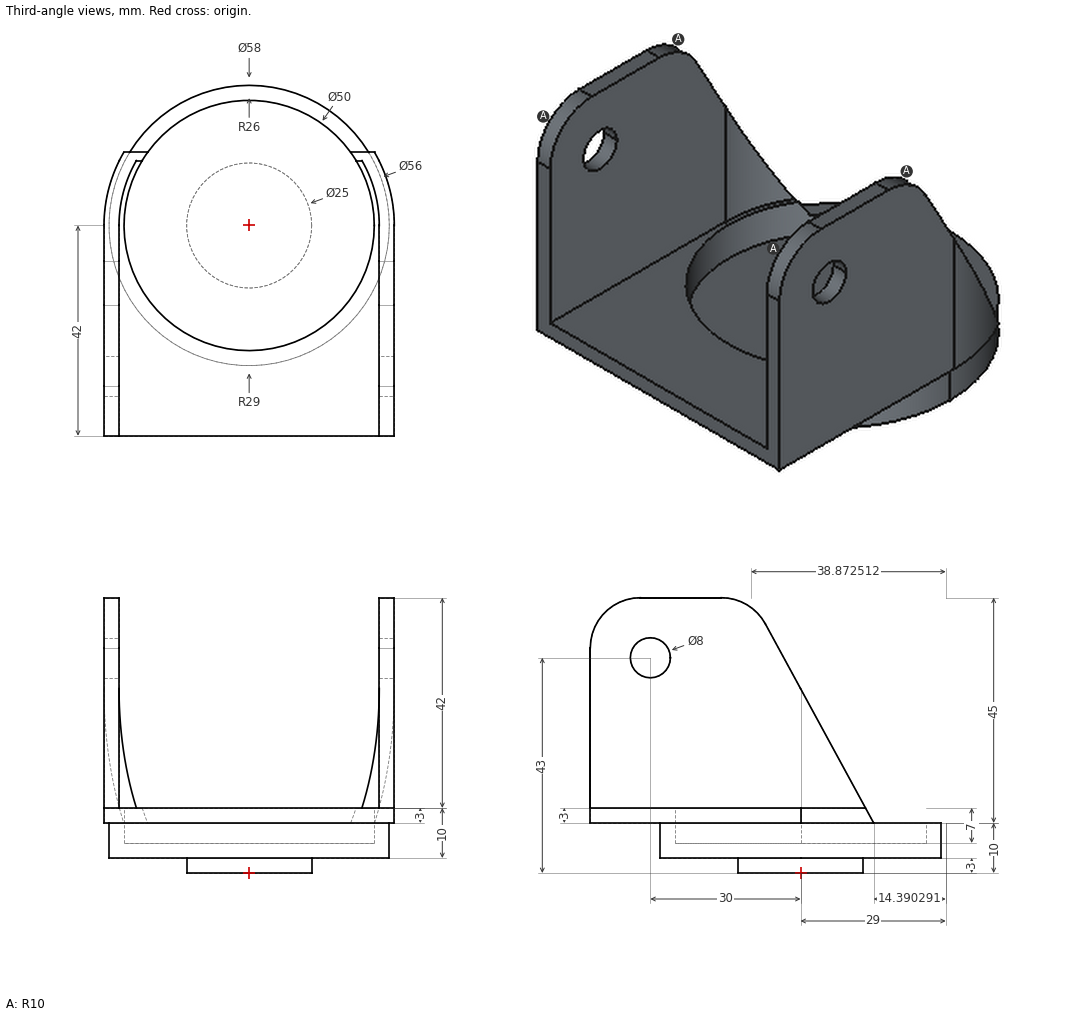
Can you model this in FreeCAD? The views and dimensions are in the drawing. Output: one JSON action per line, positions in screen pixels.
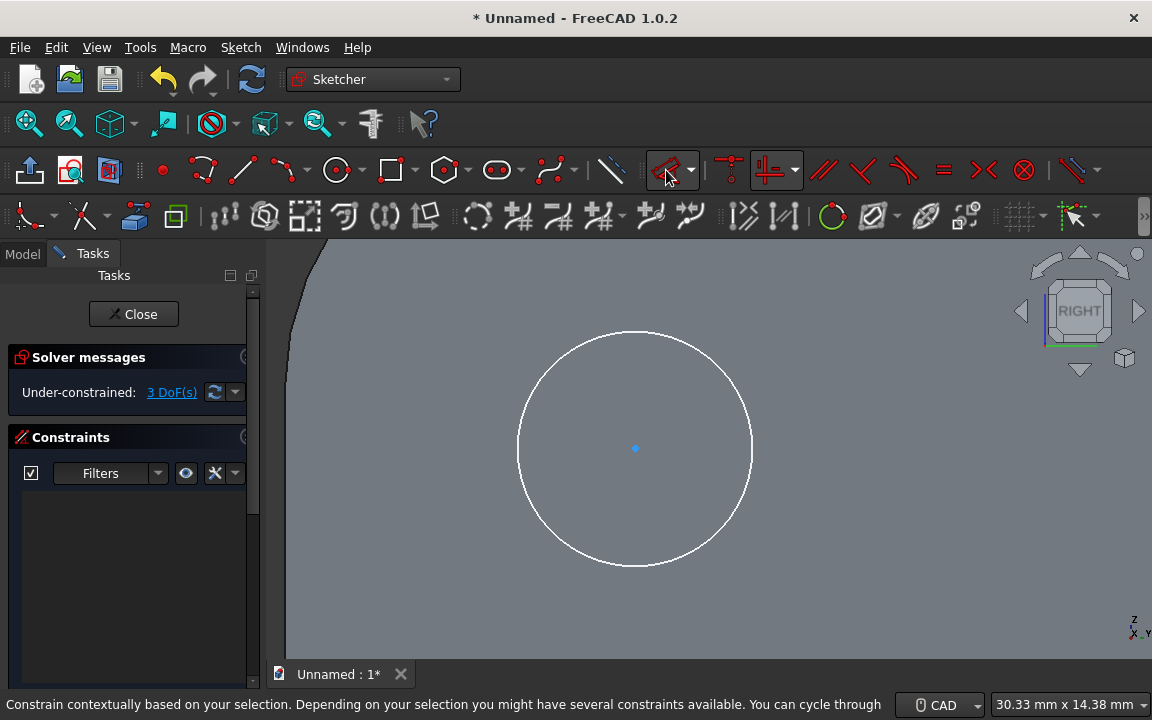
{"action": "left_click", "coordinate": [718, 366]}
{"action": "left_click", "coordinate": [741, 343]}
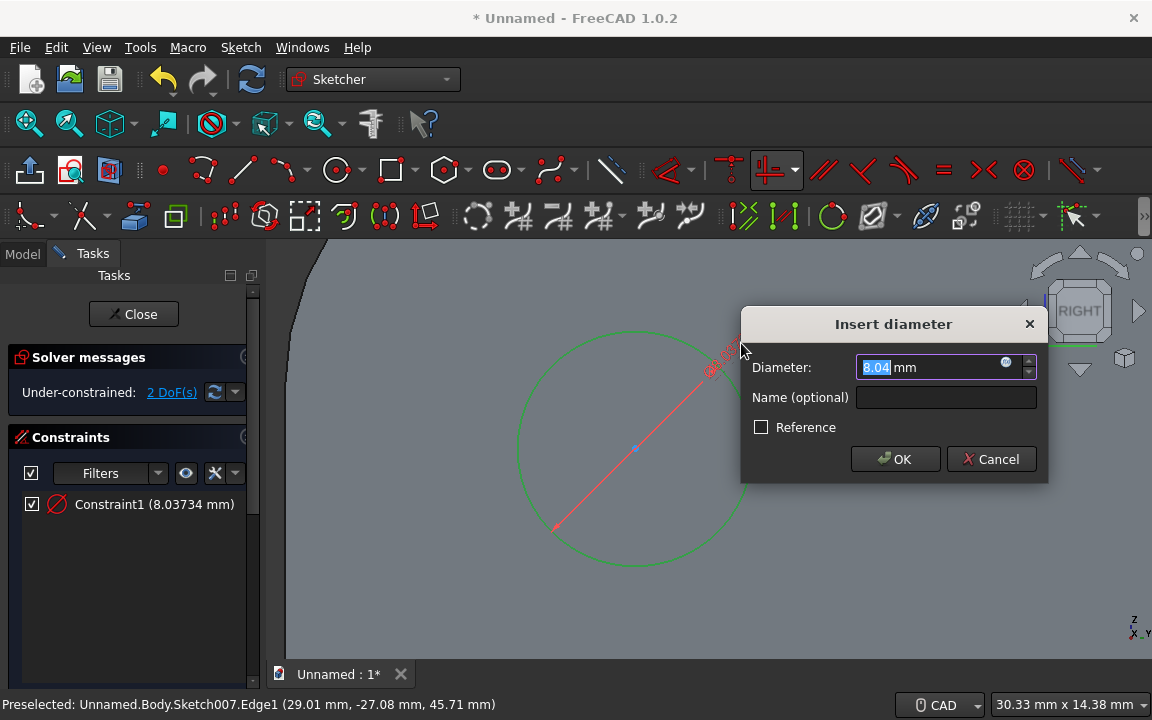
{"action": "type", "text": "8"}
{"action": "key", "text": "Return"}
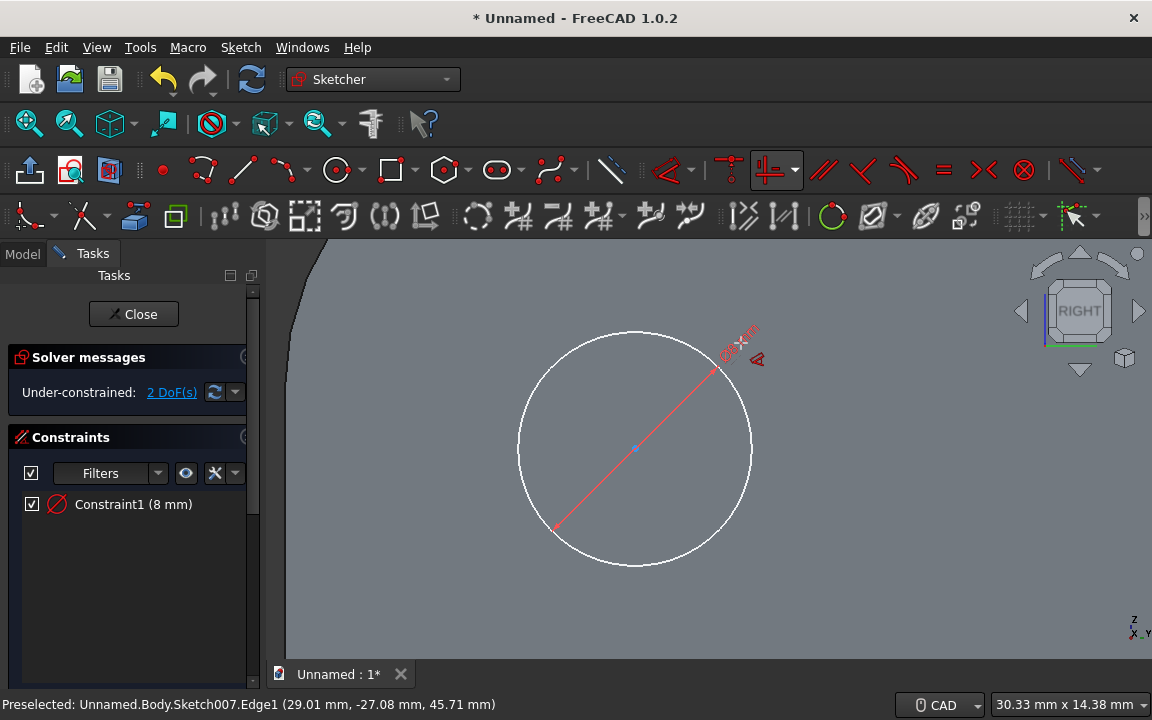
{"action": "left_click", "coordinate": [635, 449]}
{"action": "left_click", "coordinate": [811, 415]}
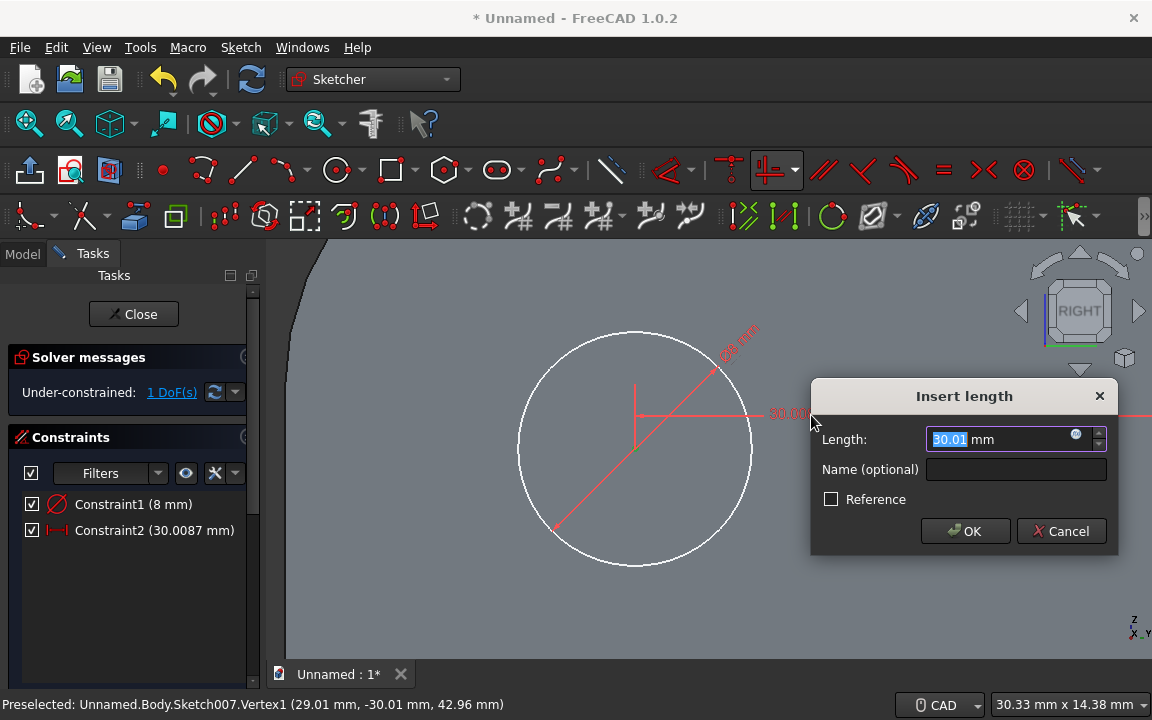
{"action": "type", "text": "30"}
{"action": "key", "text": "Return"}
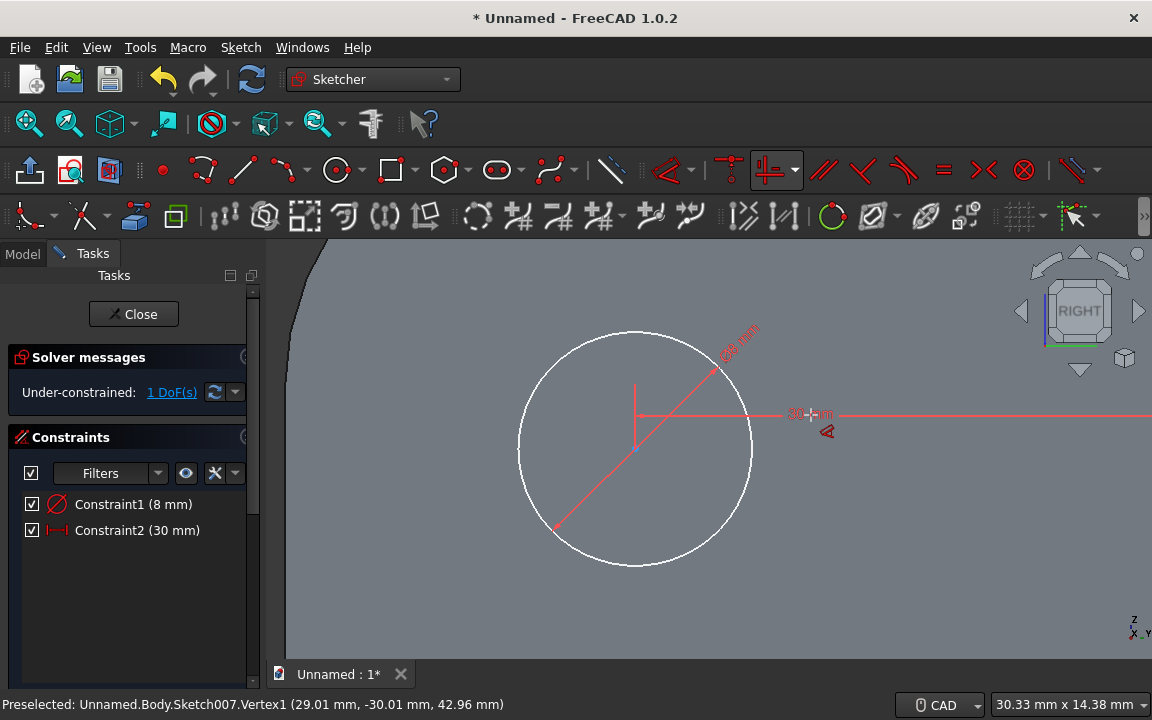
{"action": "left_click", "coordinate": [635, 449]}
{"action": "left_click", "coordinate": [601, 540]}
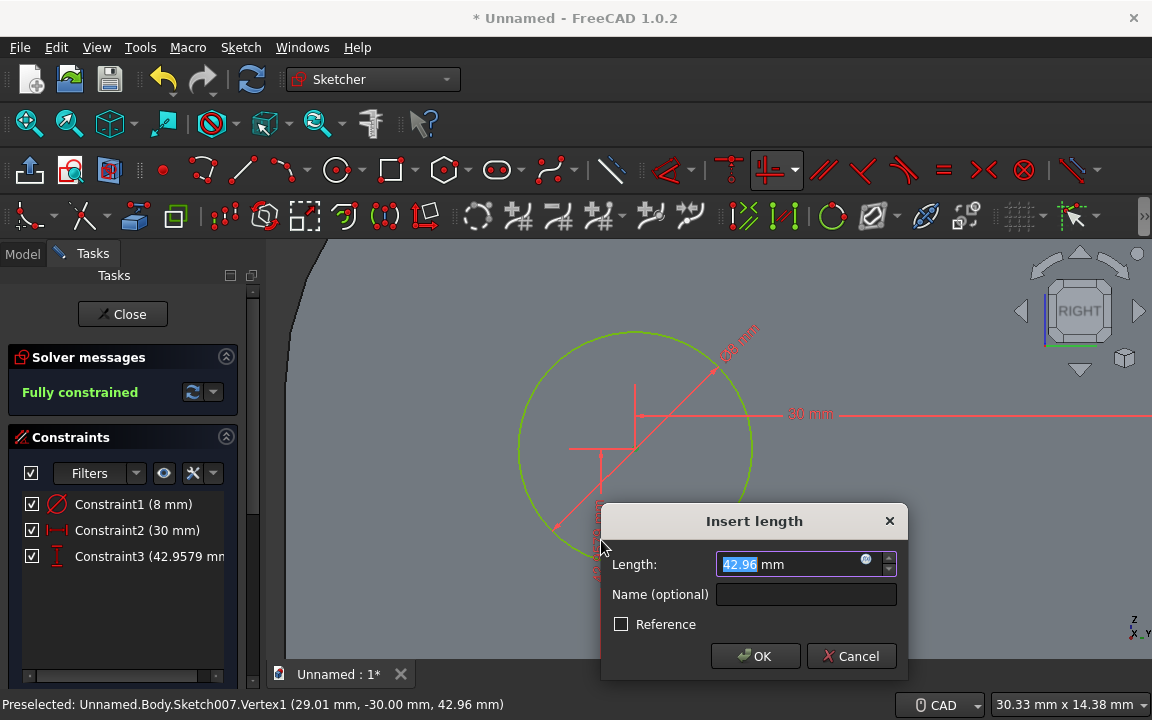
{"action": "type", "text": "43"}
{"action": "key", "text": "Return"}
{"action": "key", "text": "Escape"}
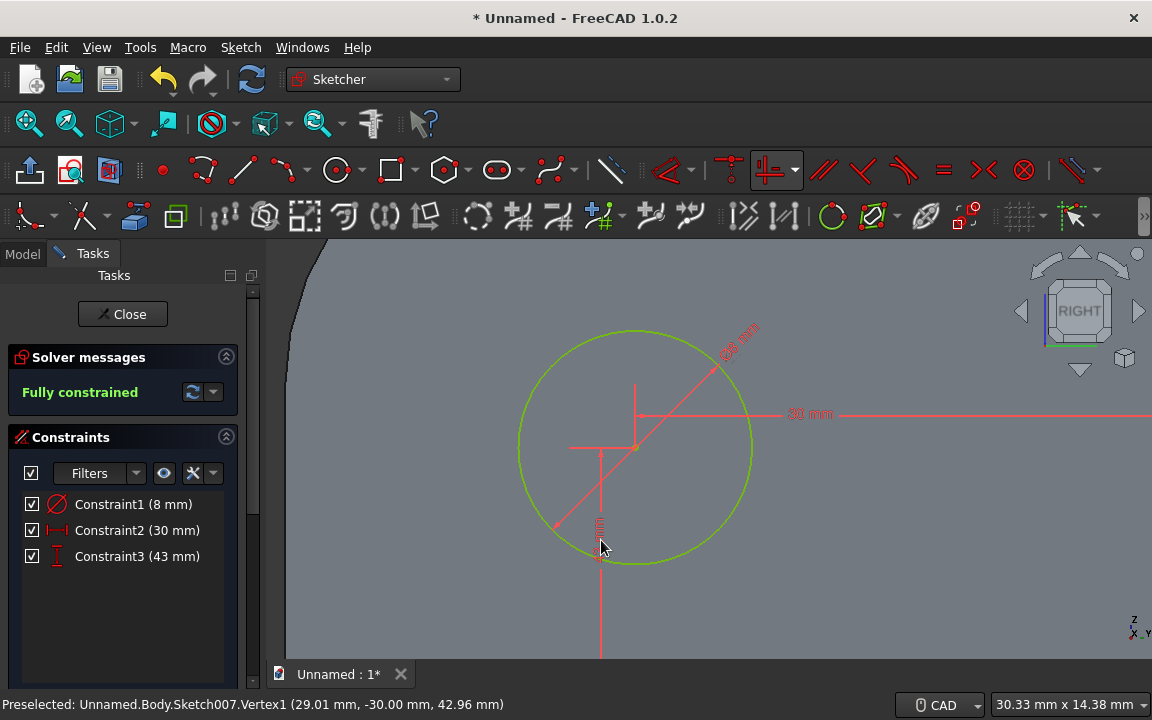
{"action": "left_click", "coordinate": [123, 314]}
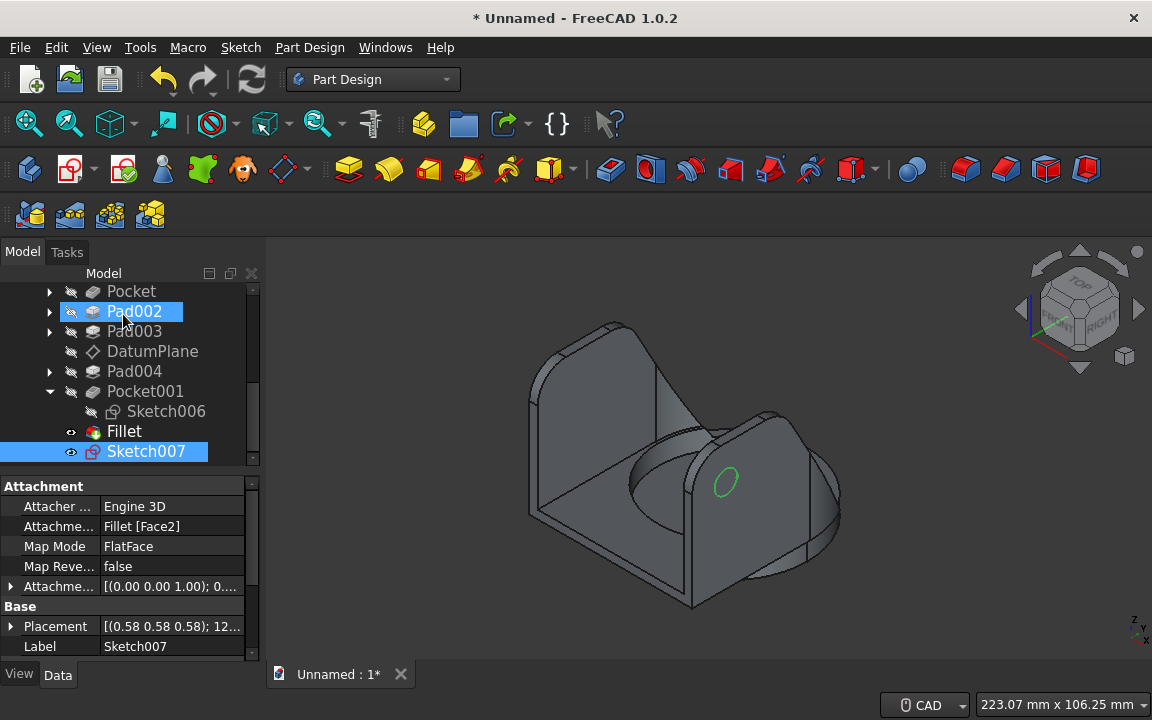
{"action": "left_click", "coordinate": [612, 170]}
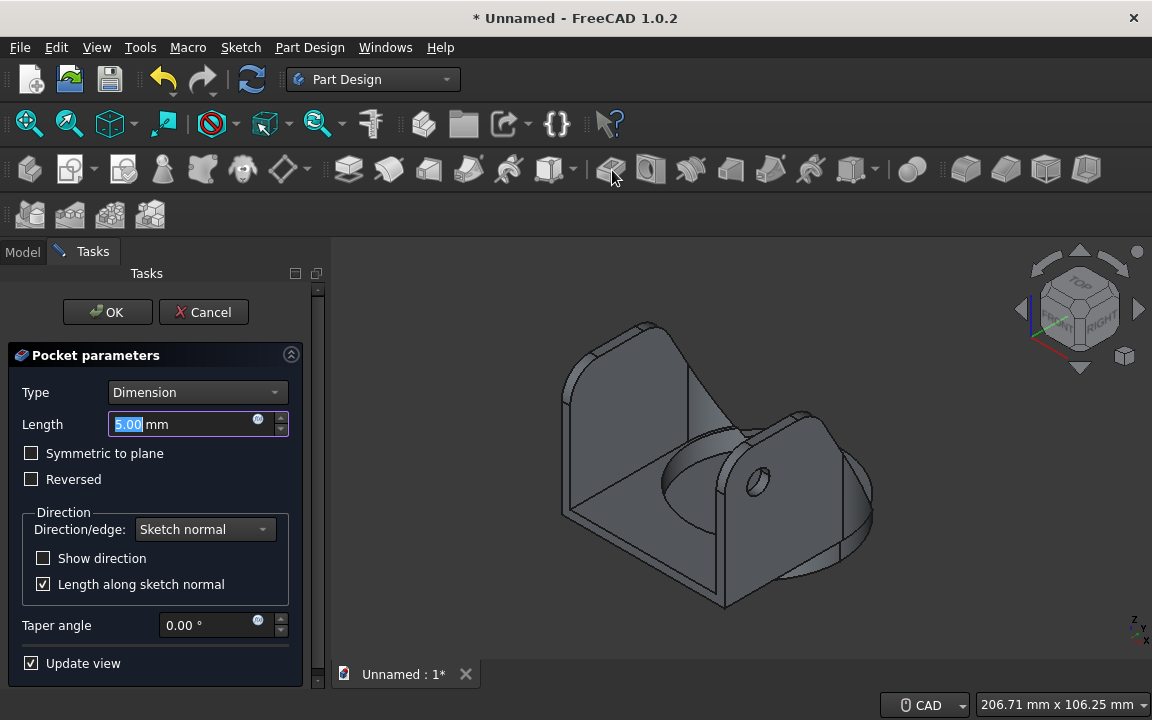
{"action": "left_click", "coordinate": [198, 392]}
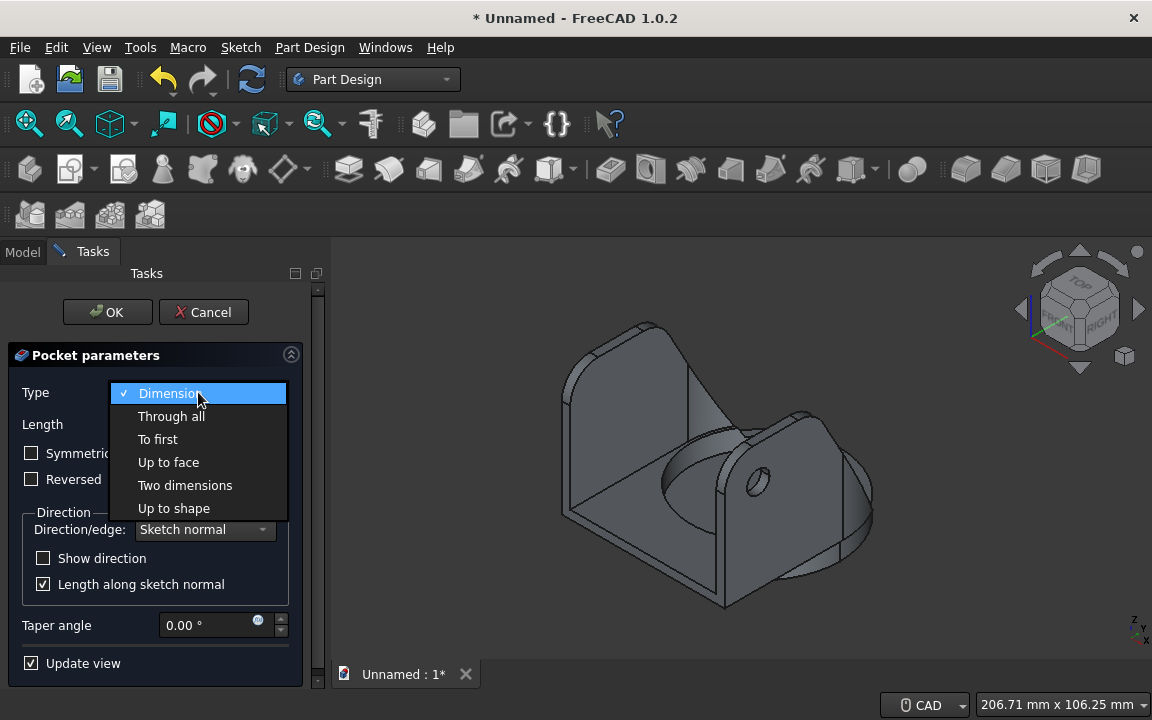
{"action": "left_click", "coordinate": [198, 416]}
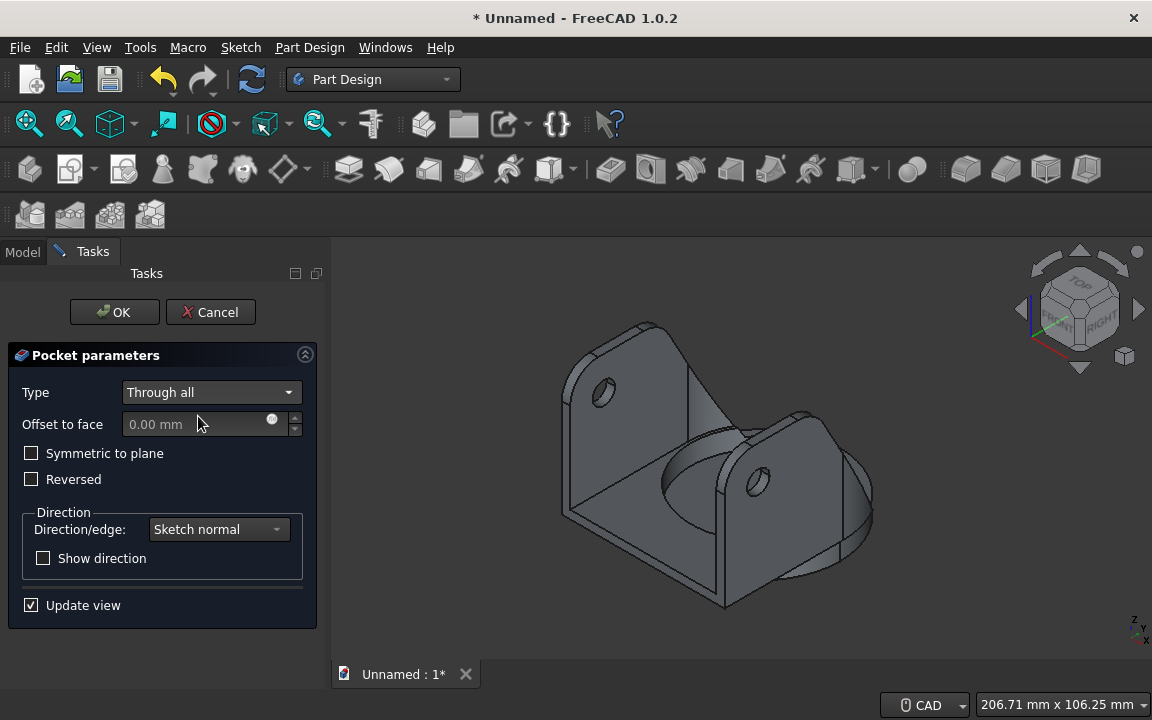
{"action": "left_click", "coordinate": [115, 312]}